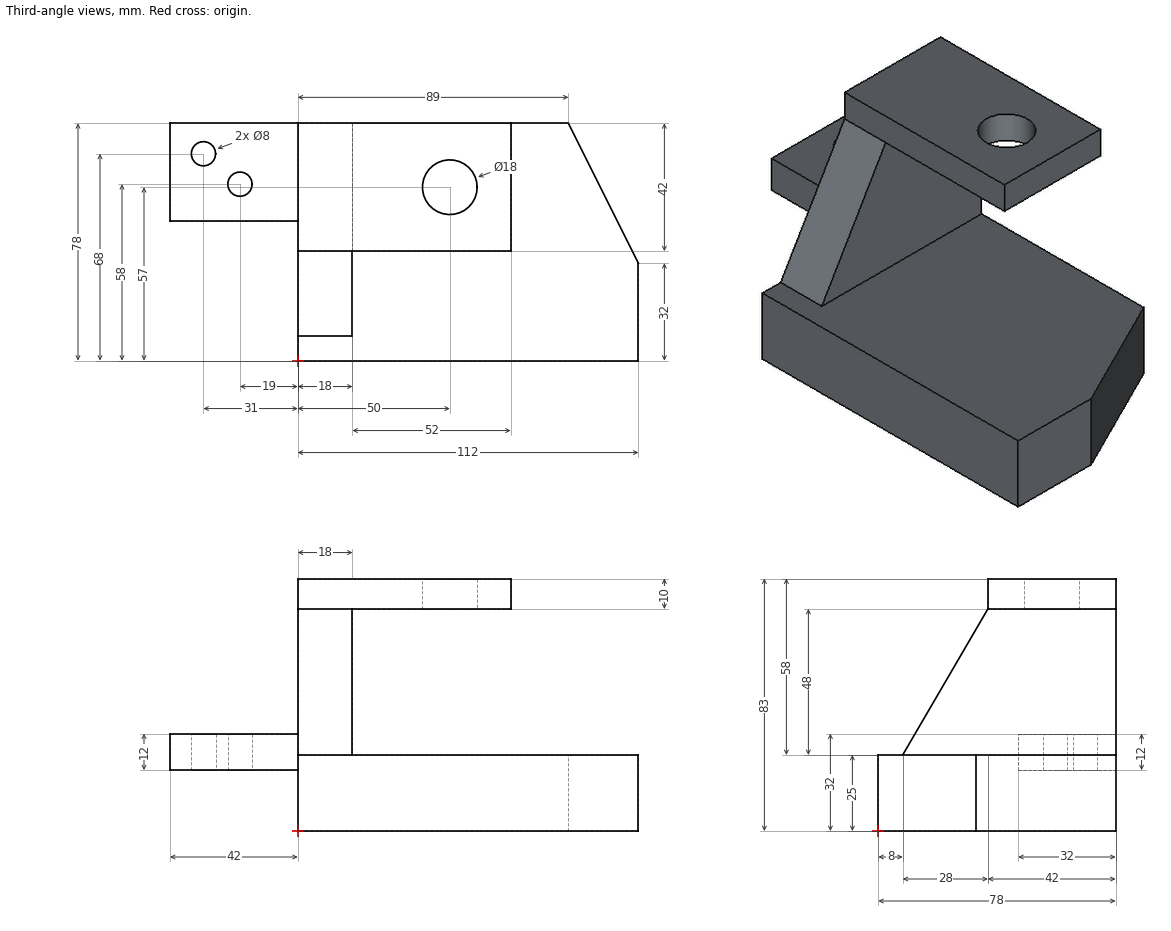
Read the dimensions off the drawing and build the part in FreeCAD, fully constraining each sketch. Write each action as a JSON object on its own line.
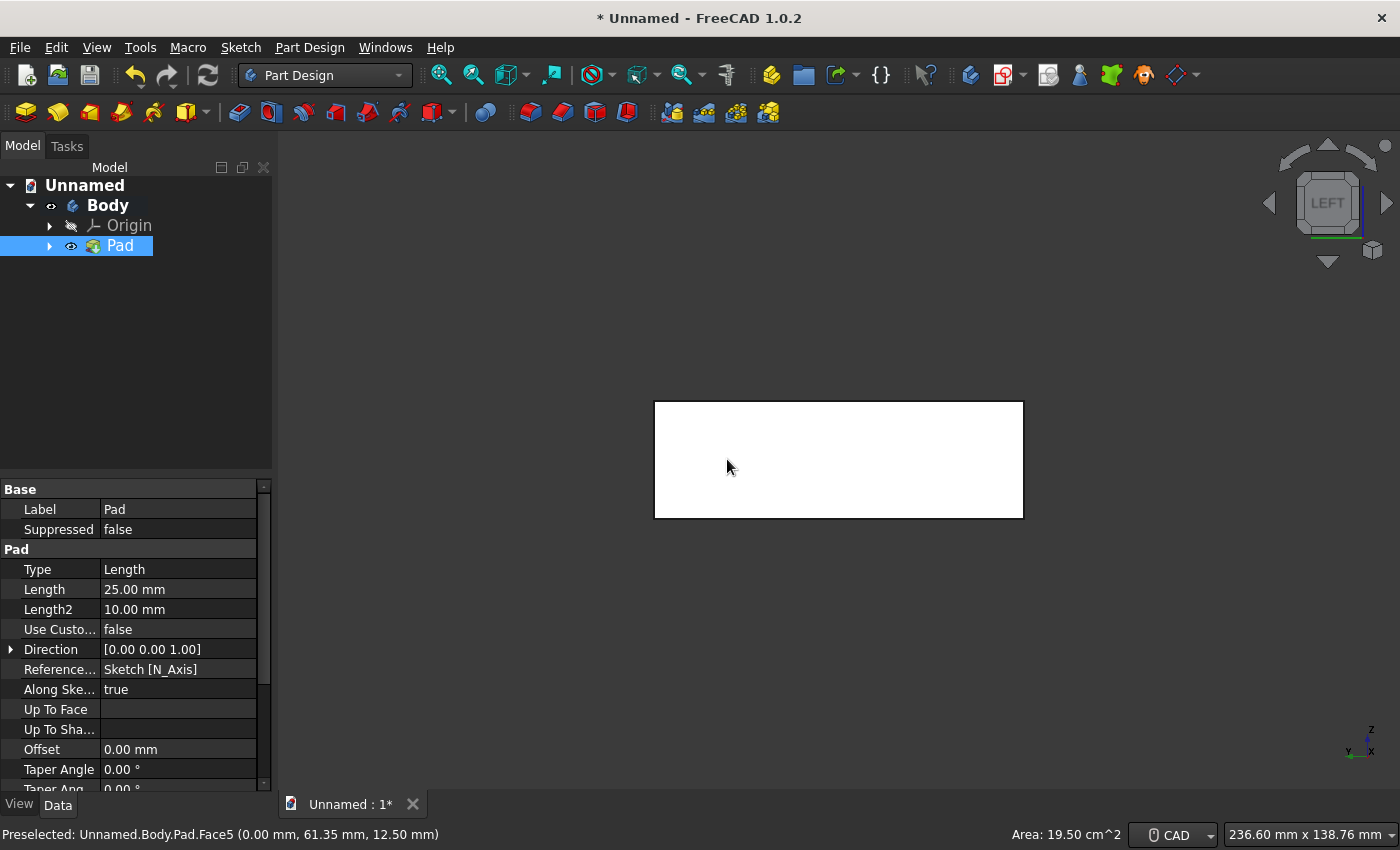
{"action": "left_click", "coordinate": [1004, 76]}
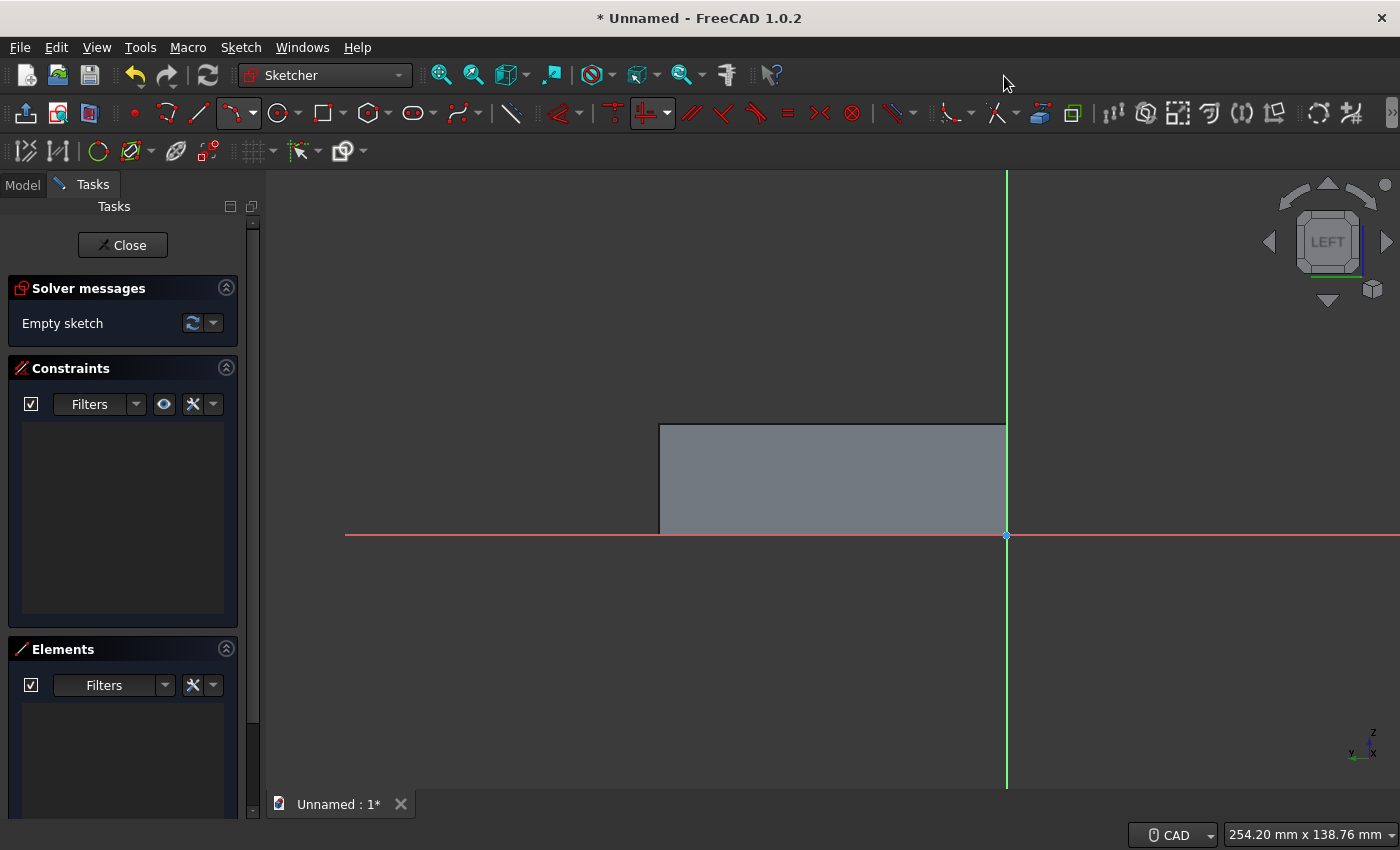
{"action": "scroll", "coordinate": [455, 761], "scroll_direction": "down", "scroll_amount": 1}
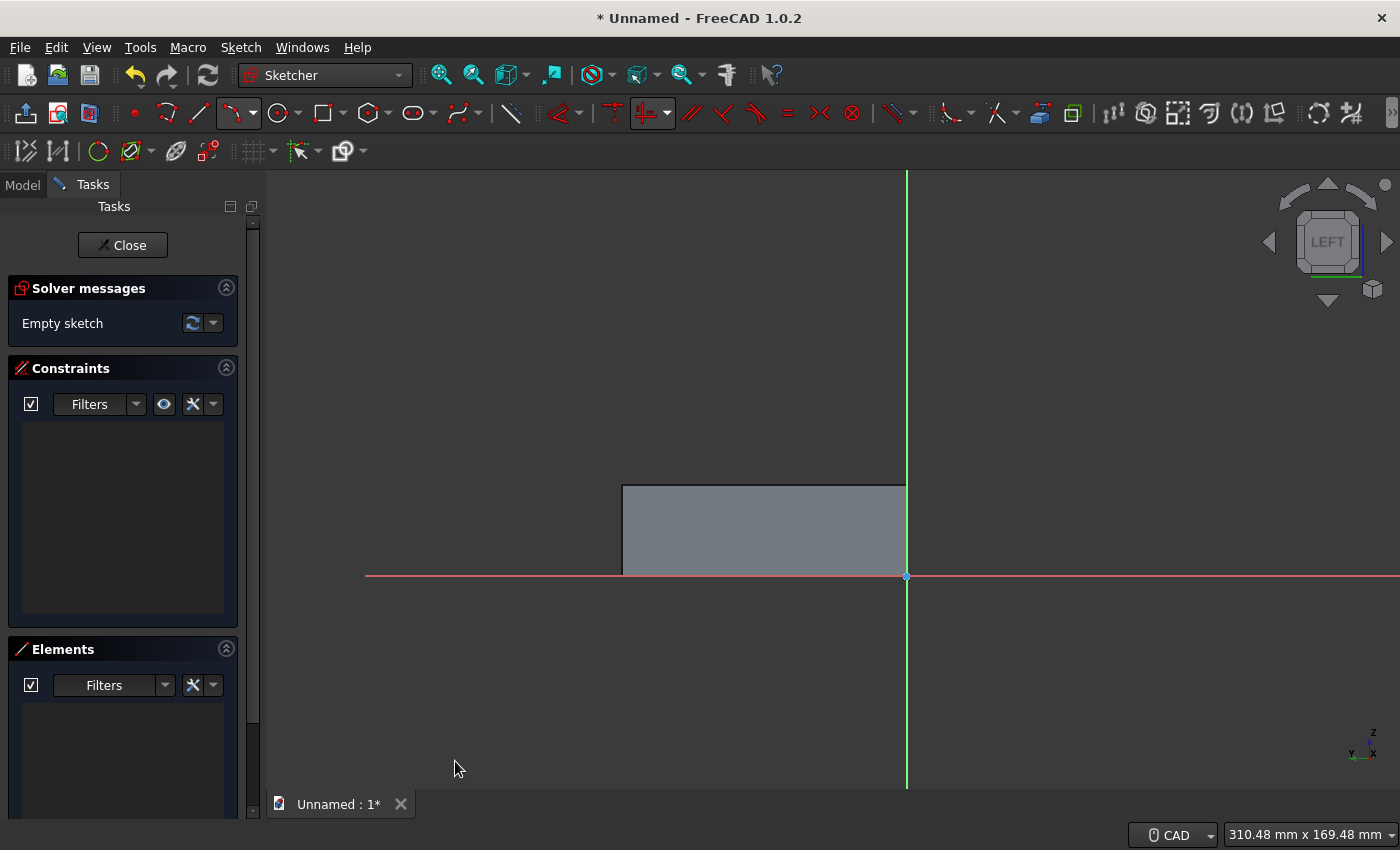
{"action": "left_click", "coordinate": [324, 114]}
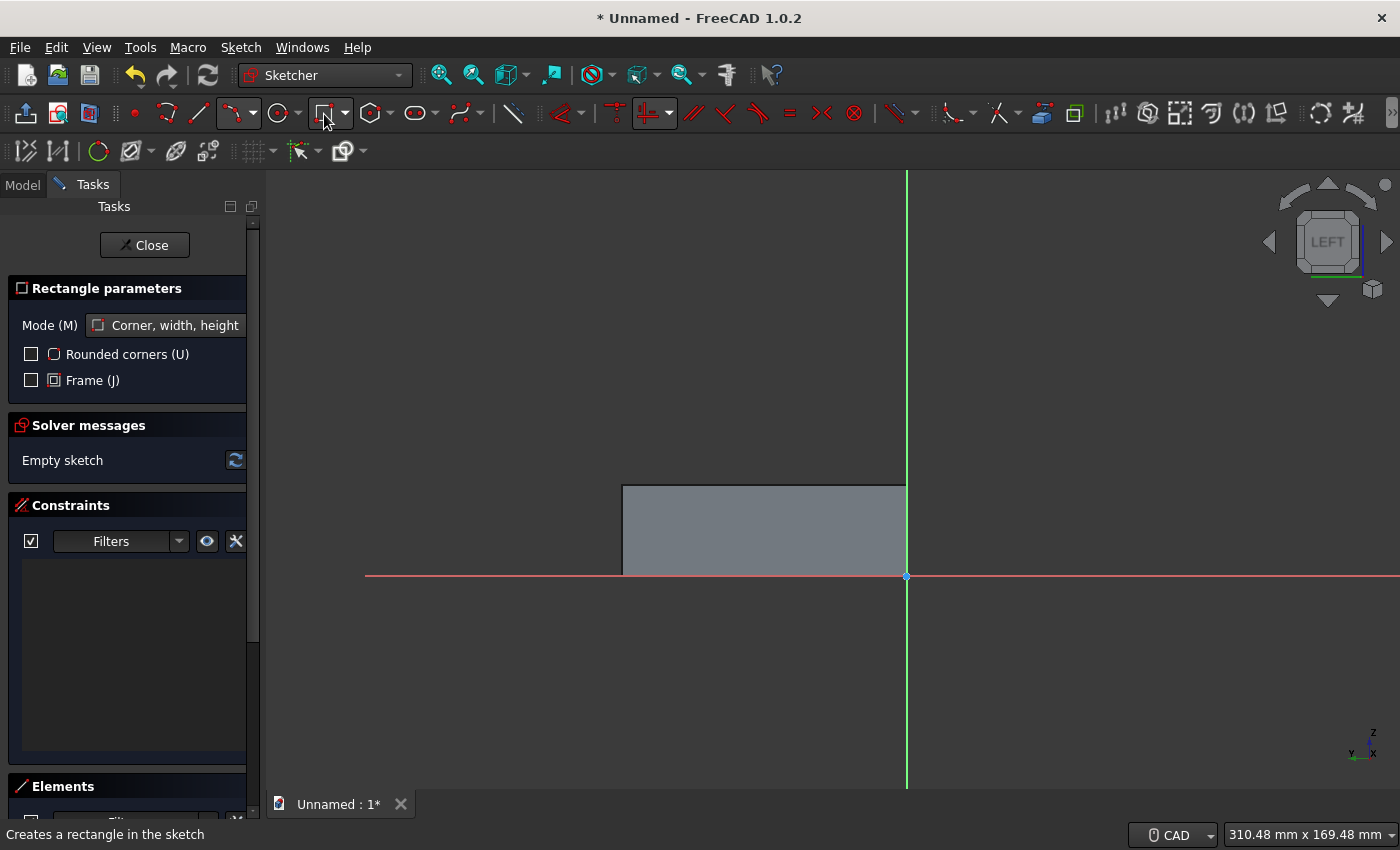
{"action": "left_click", "coordinate": [622, 273]}
{"action": "mouse_move", "coordinate": [775, 485]}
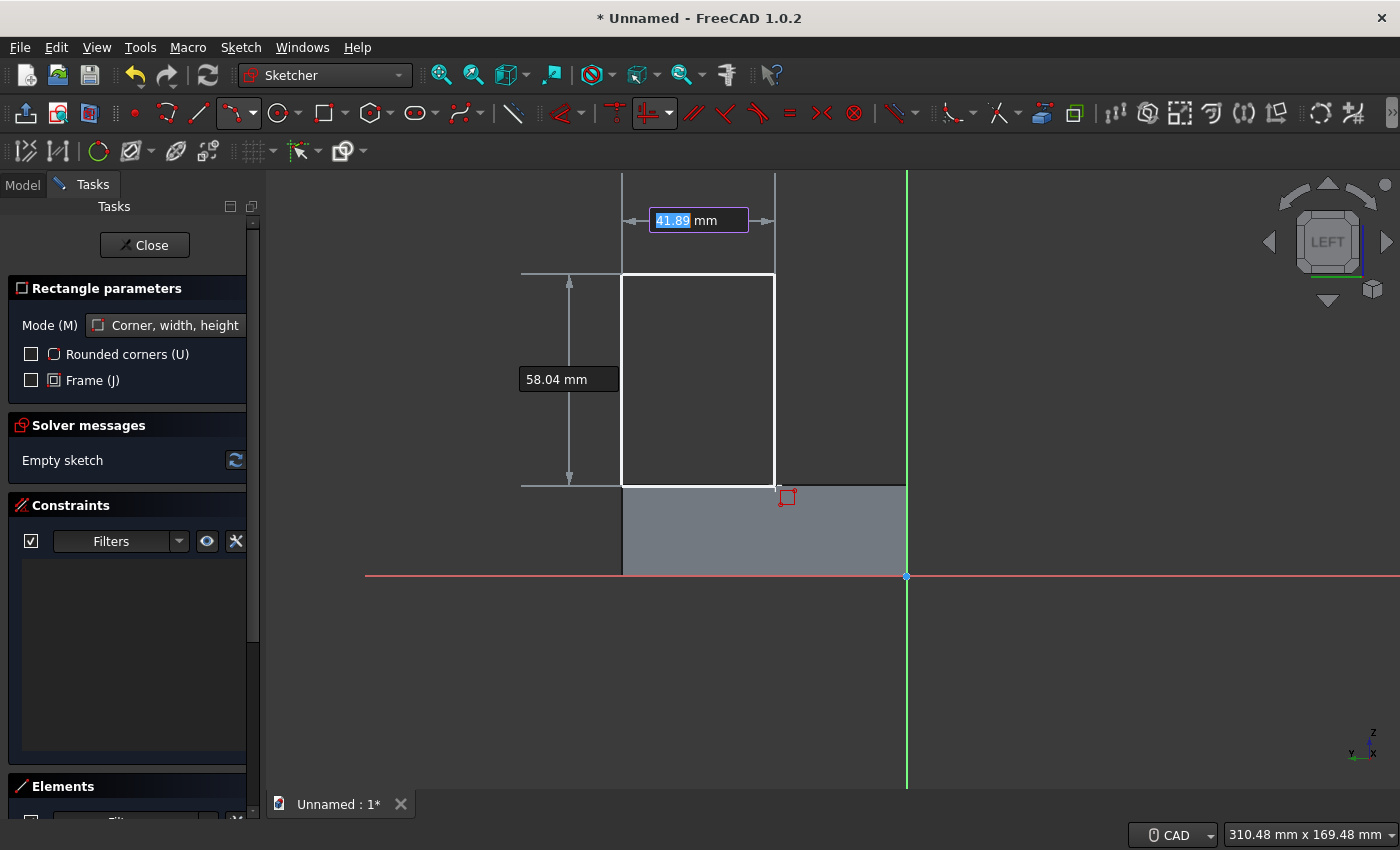
{"action": "type", "text": "42"}
{"action": "key", "text": "Tab"}
{"action": "type", "text": "58"}
{"action": "key", "text": "Return"}
{"action": "key", "text": "Escape"}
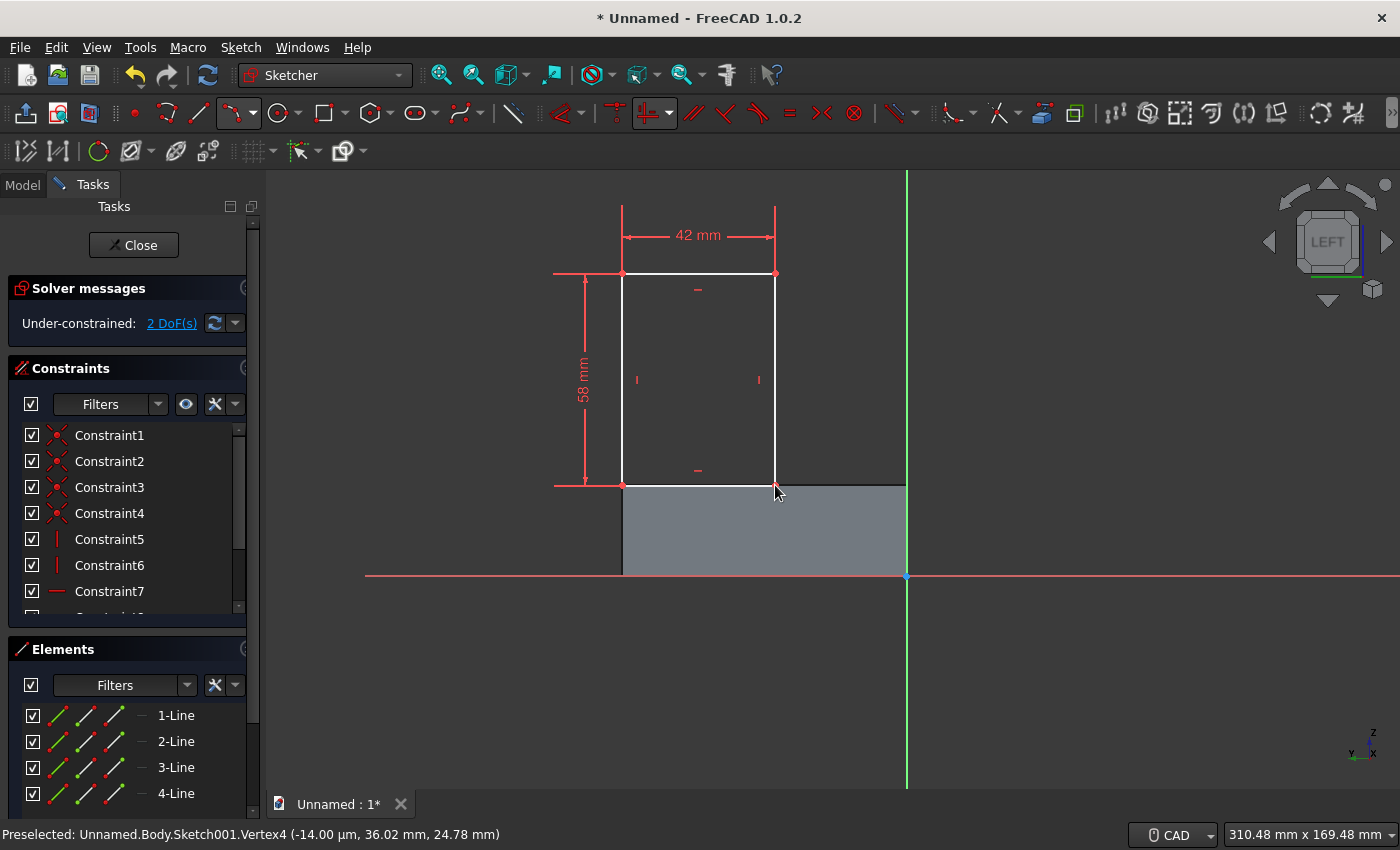
{"action": "key", "text": "d"}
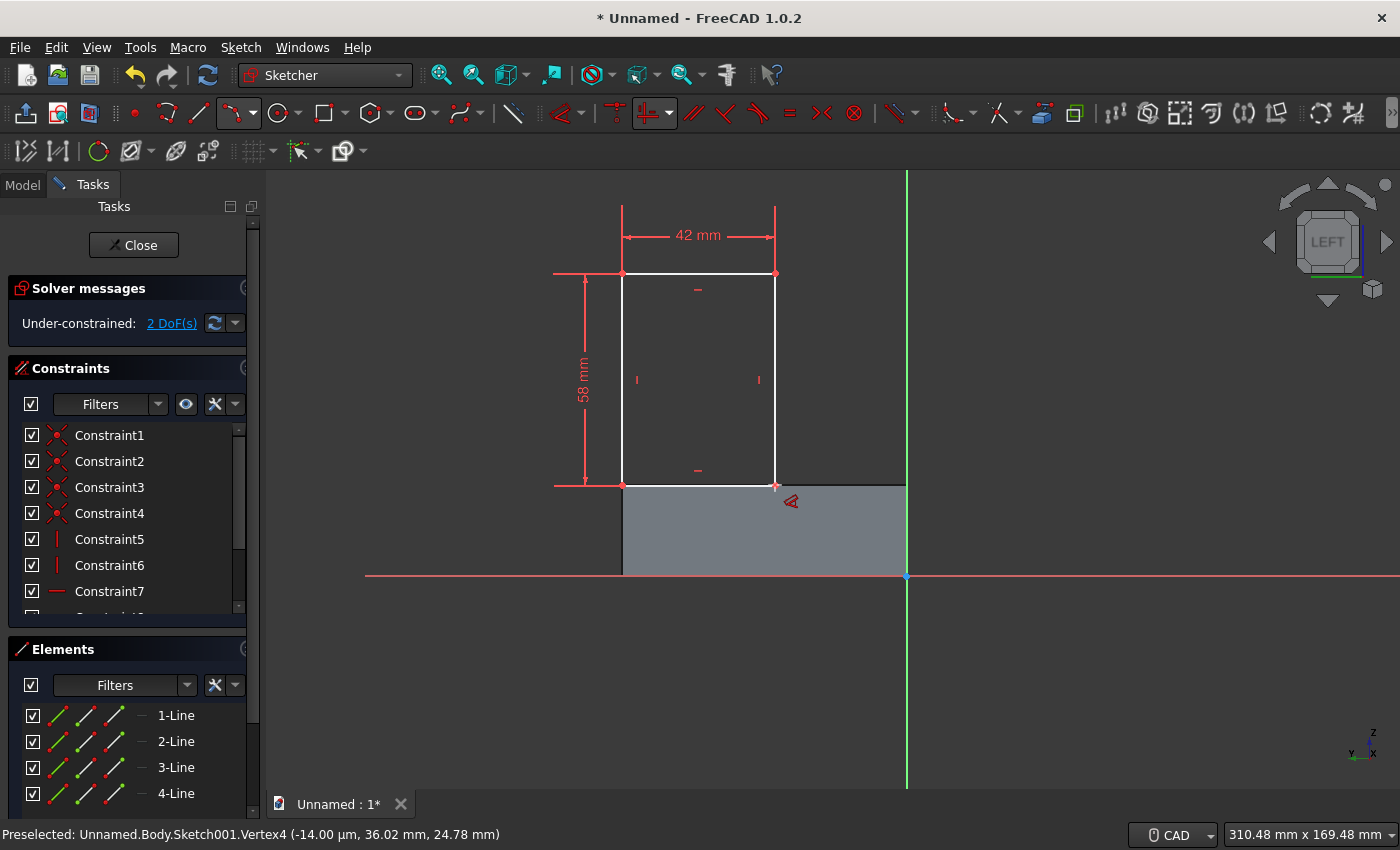
{"action": "left_click", "coordinate": [622, 274]}
{"action": "left_click", "coordinate": [764, 610]}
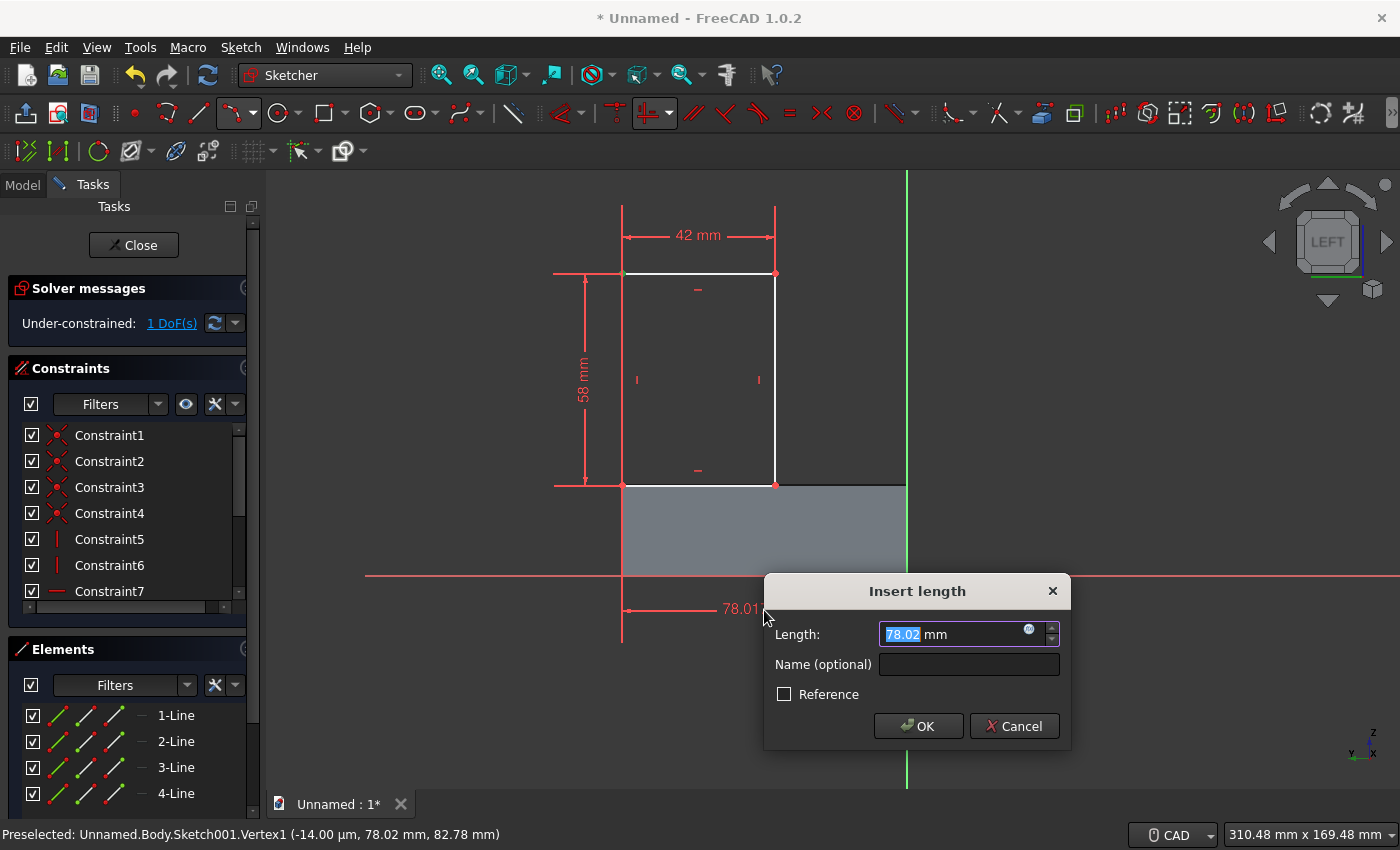
{"action": "type", "text": "78"}
{"action": "key", "text": "Return"}